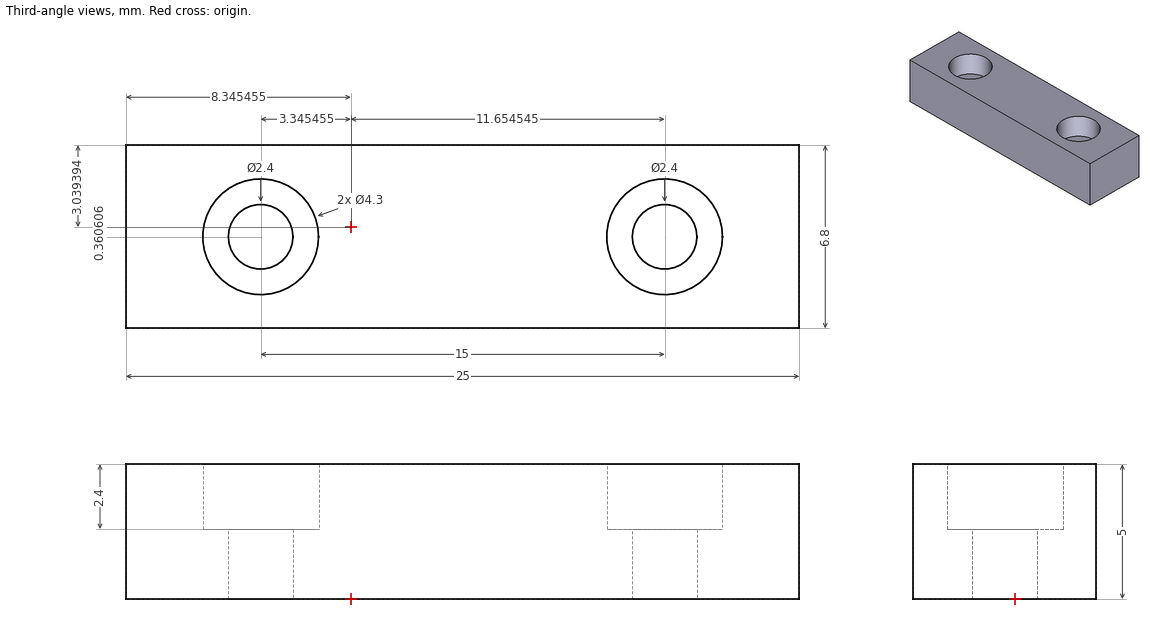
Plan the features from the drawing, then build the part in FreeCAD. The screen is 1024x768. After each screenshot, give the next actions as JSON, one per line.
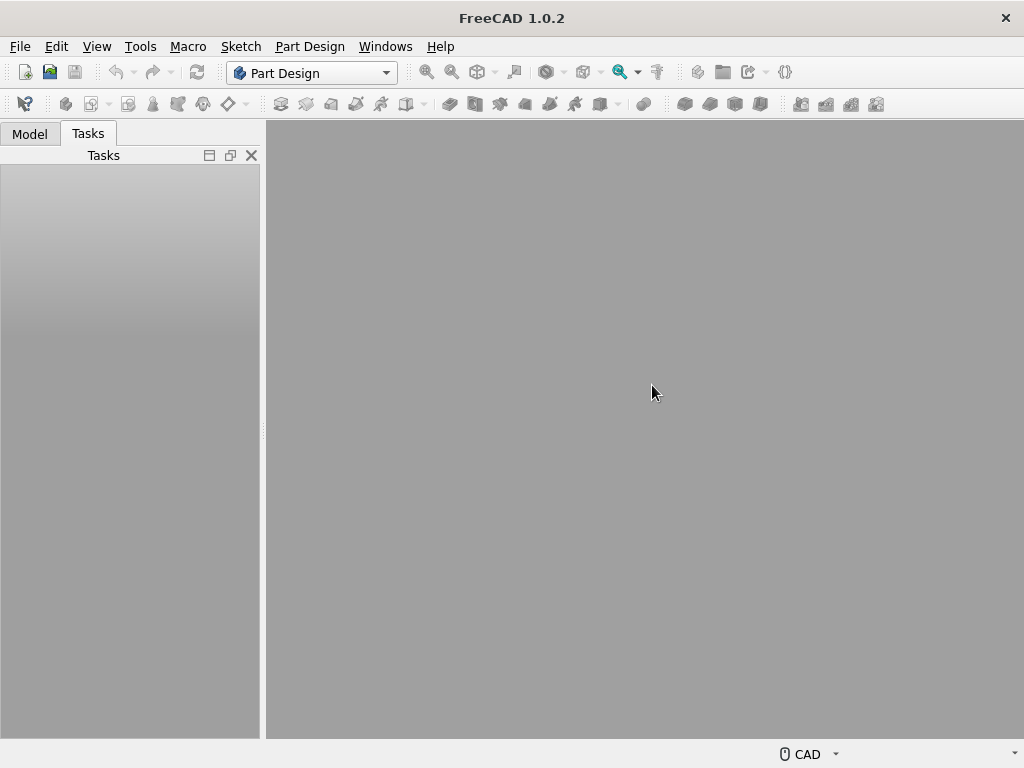
{"action": "left_click", "coordinate": [25, 72]}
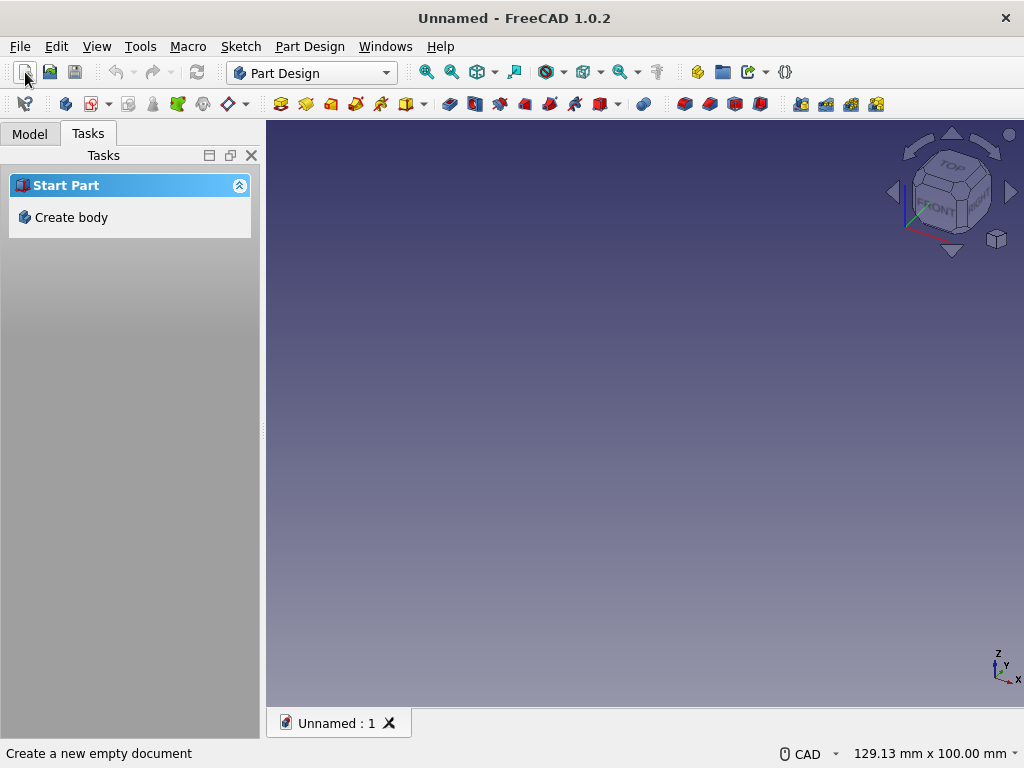
{"action": "left_click", "coordinate": [90, 104]}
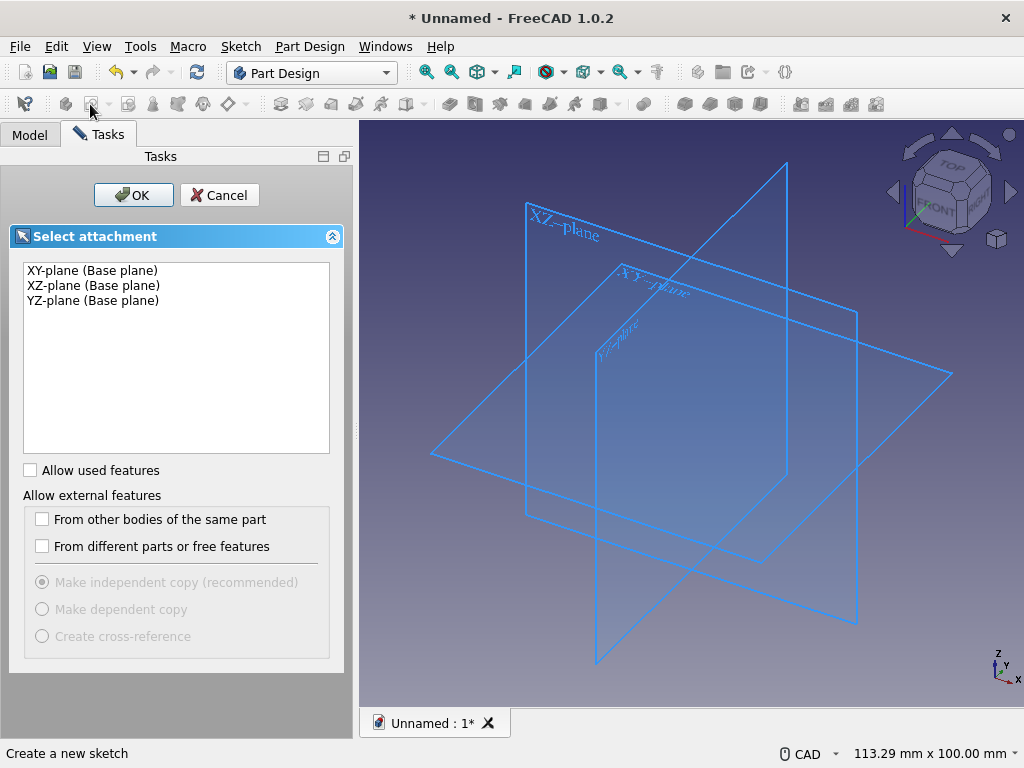
{"action": "left_click", "coordinate": [84, 270]}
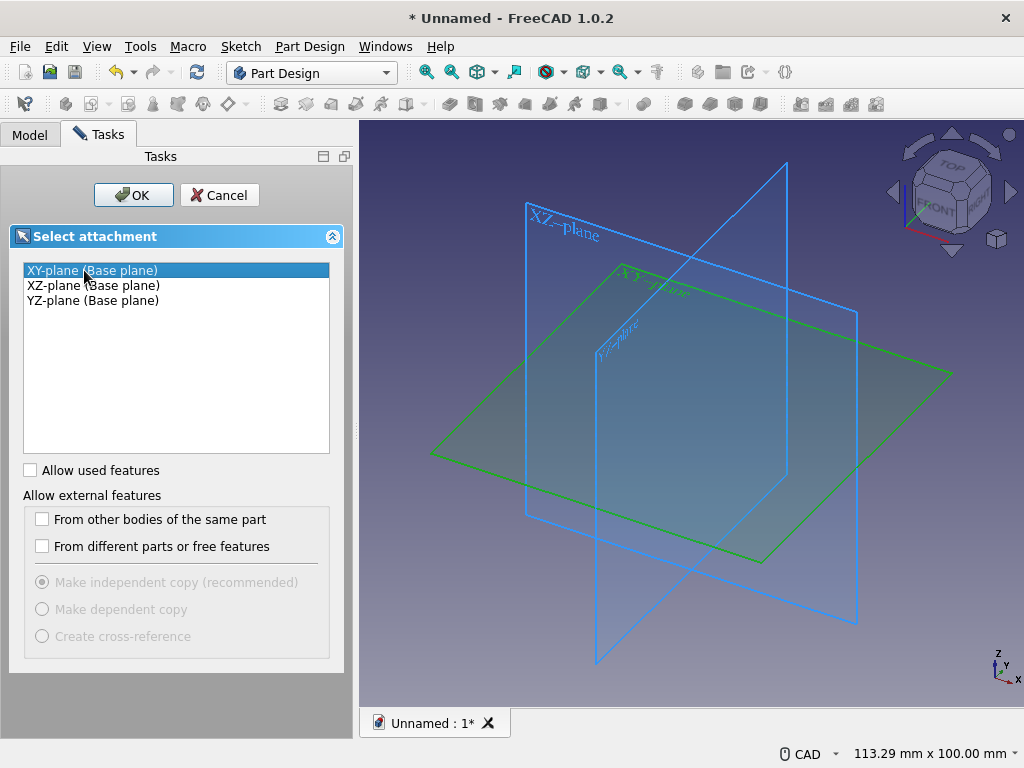
{"action": "left_click", "coordinate": [134, 195]}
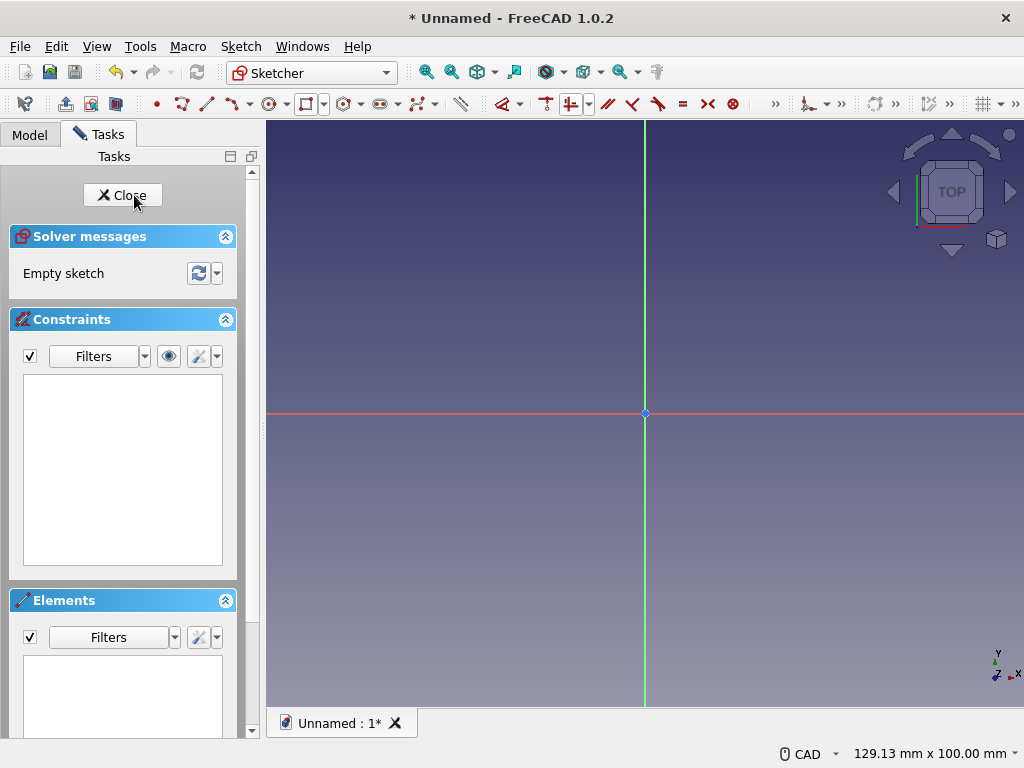
{"action": "scroll", "coordinate": [723, 417], "scroll_direction": "up", "scroll_amount": 5}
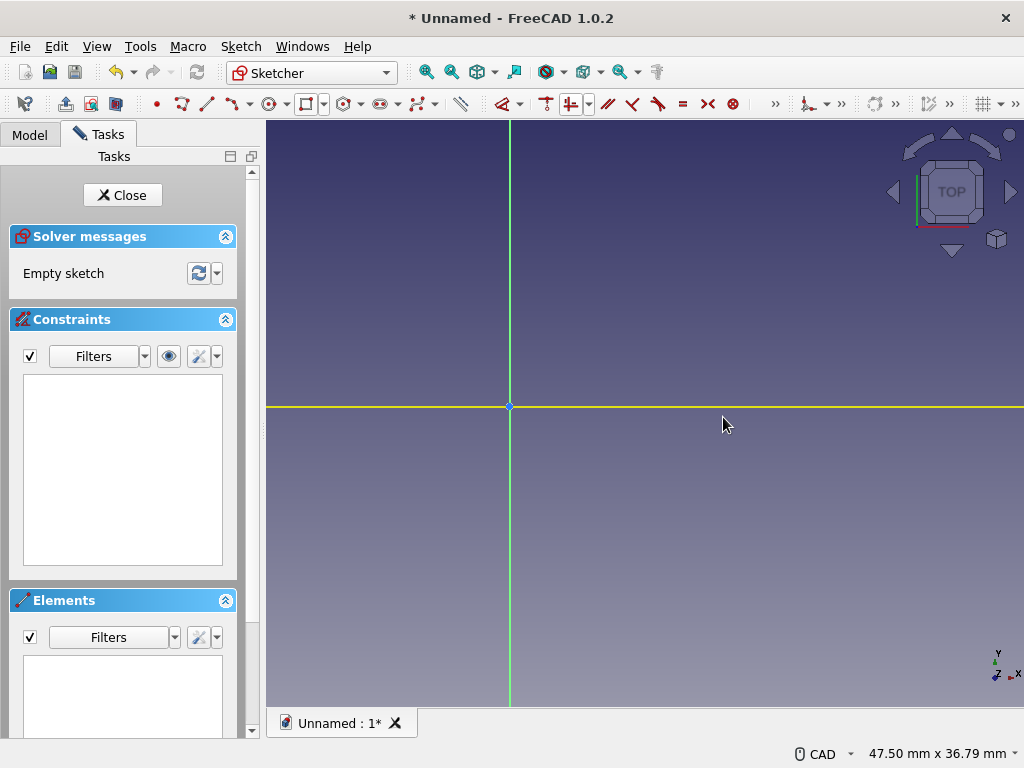
{"action": "left_click", "coordinate": [306, 104]}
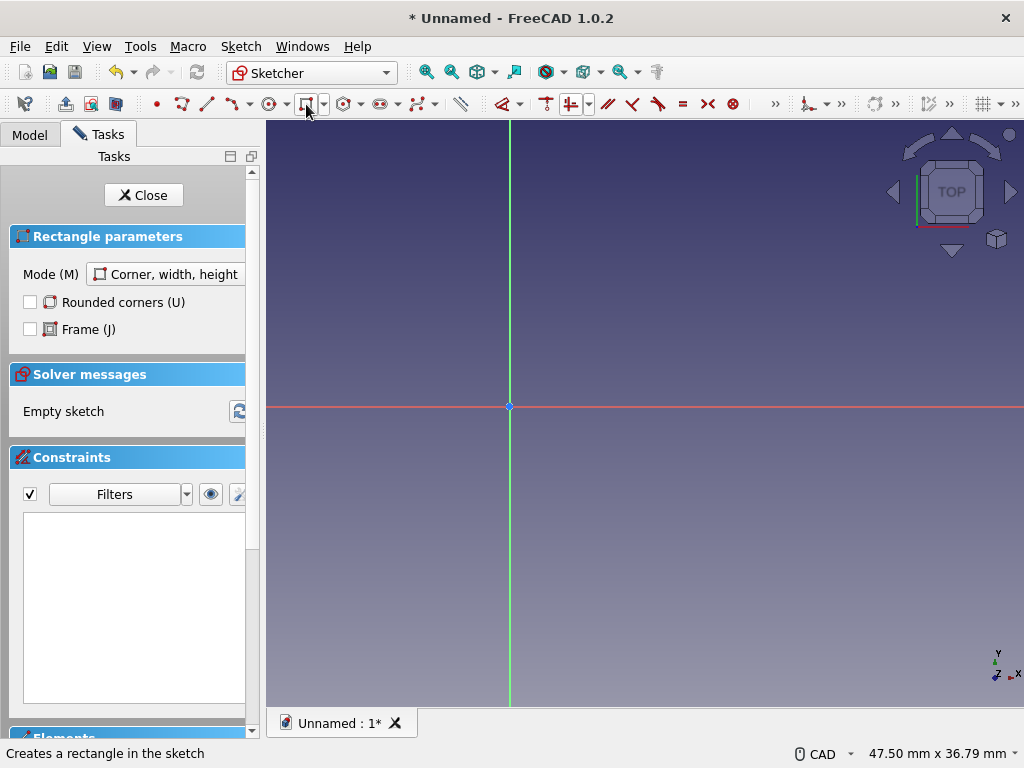
{"action": "left_click", "coordinate": [377, 358]}
{"action": "mouse_move", "coordinate": [776, 467]}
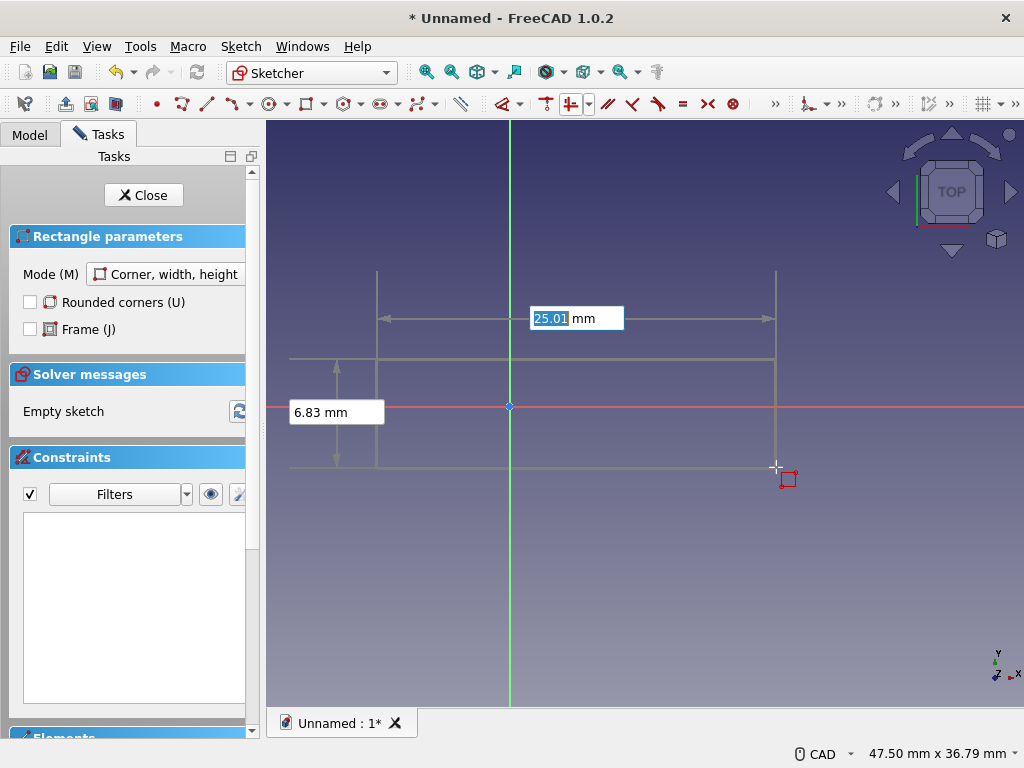
{"action": "type", "text": "25"}
{"action": "key", "text": "Tab"}
{"action": "type", "text": "6.8"}
{"action": "key", "text": "Return"}
{"action": "key", "text": "Escape"}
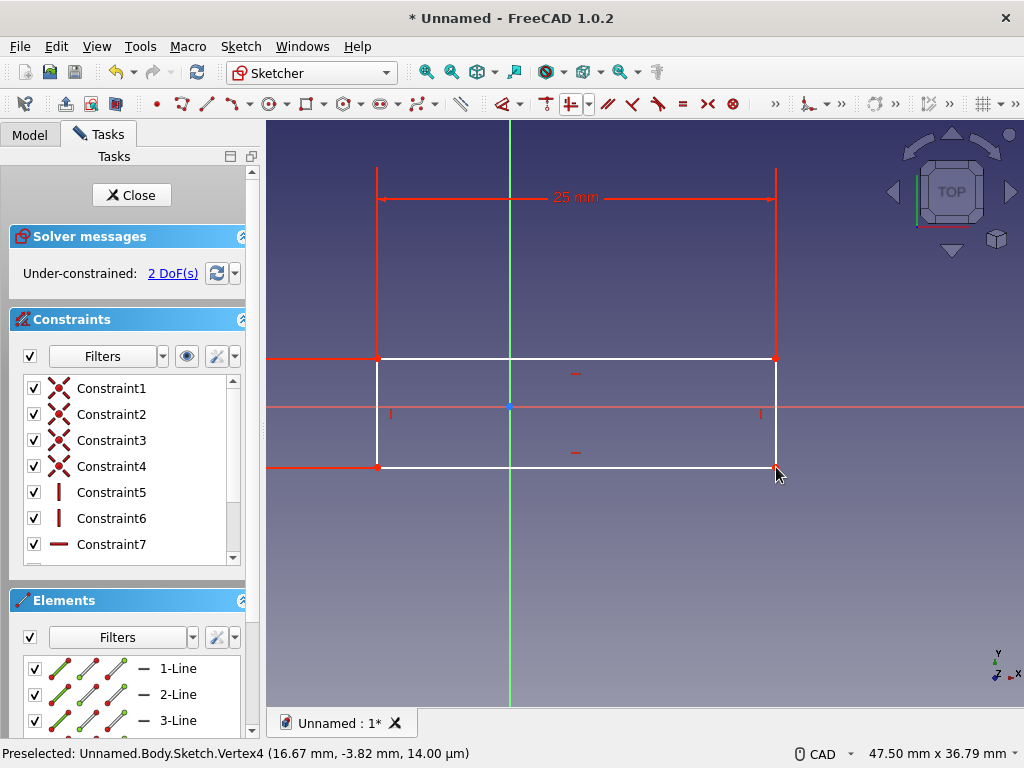
{"action": "left_click", "coordinate": [502, 104]}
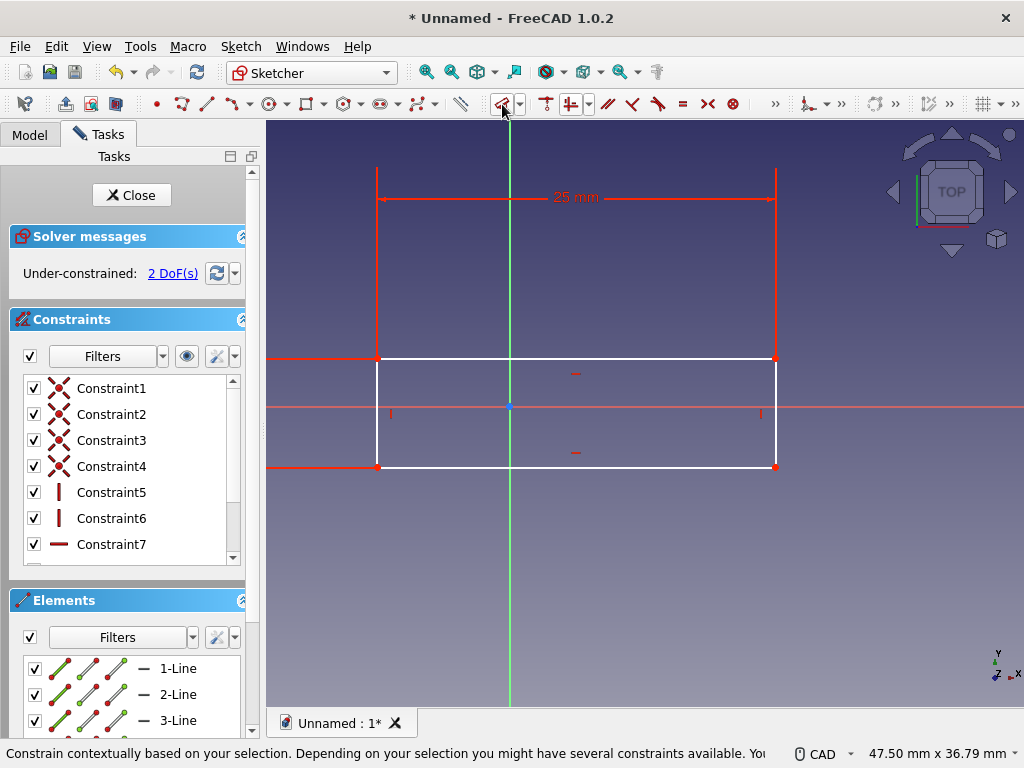
{"action": "left_click", "coordinate": [377, 359]}
{"action": "left_click", "coordinate": [443, 325]}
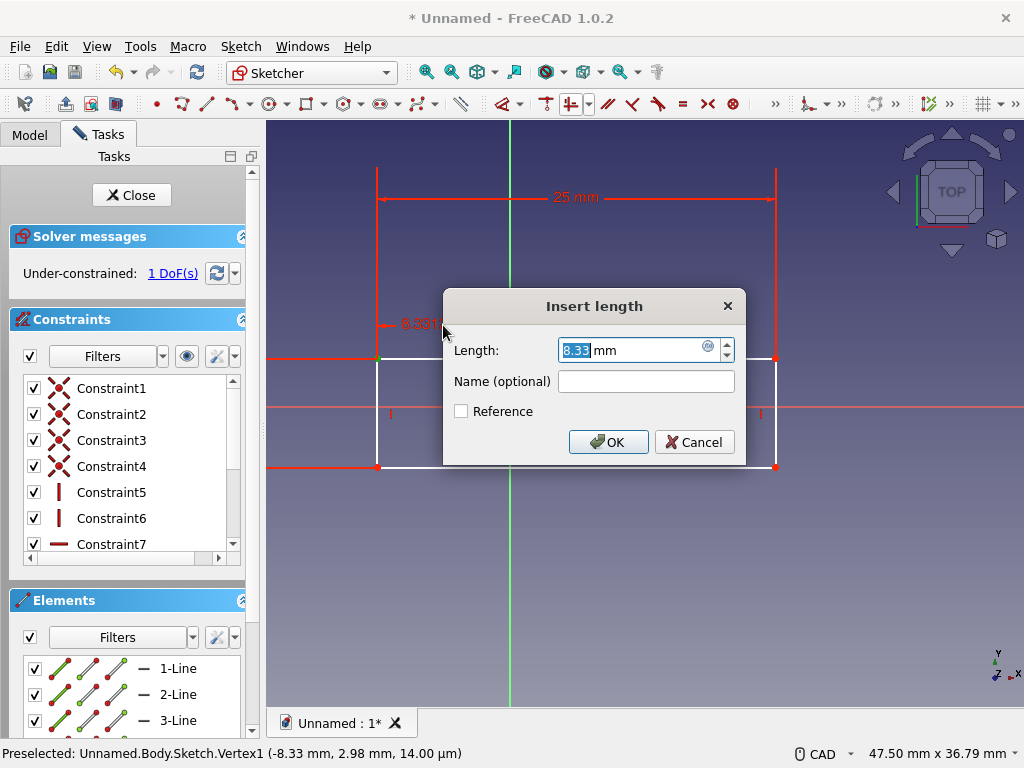
{"action": "type", "text": "8.345455"}
{"action": "key", "text": "Return"}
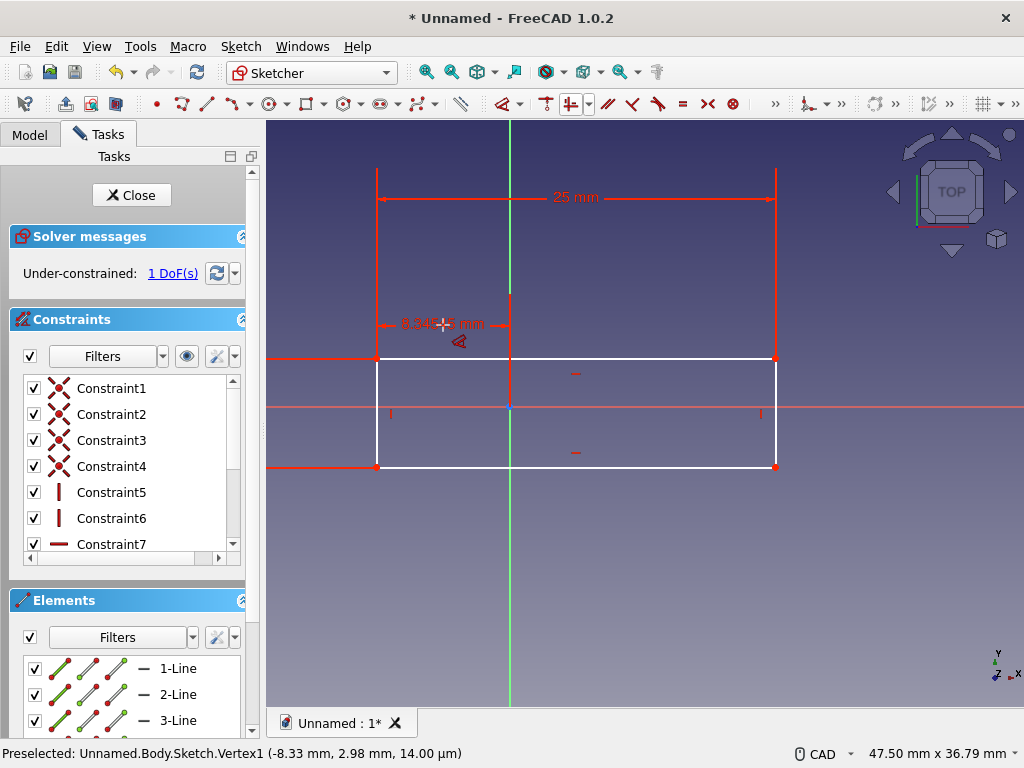
{"action": "left_click", "coordinate": [377, 359]}
{"action": "left_click", "coordinate": [343, 383]}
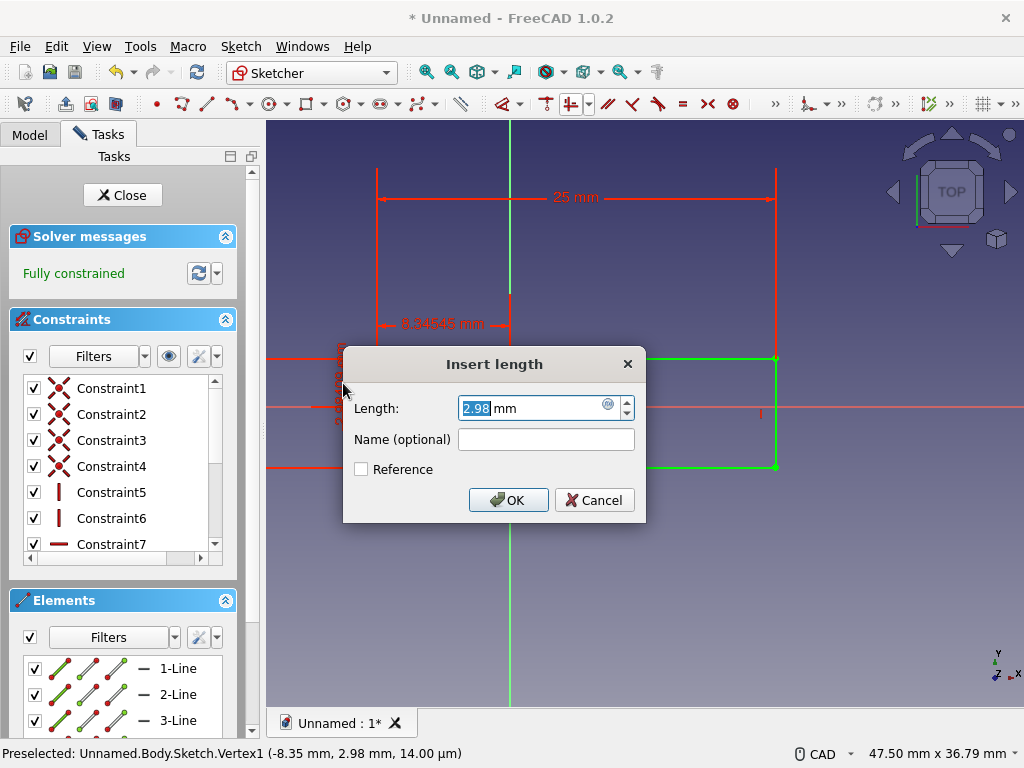
{"action": "type", "text": "3.039394"}
{"action": "key", "text": "Return"}
{"action": "key", "text": "Escape"}